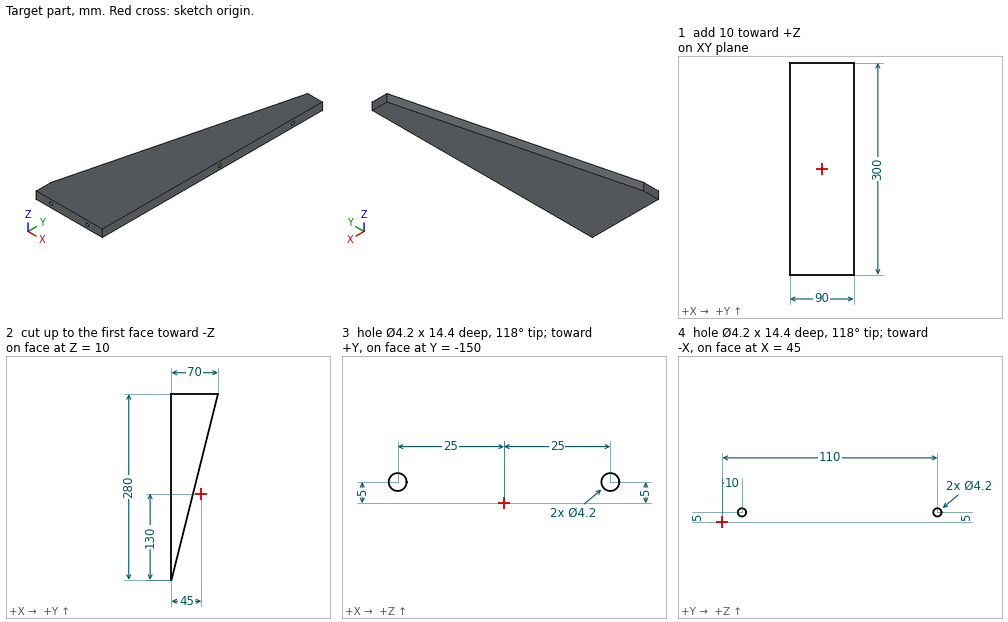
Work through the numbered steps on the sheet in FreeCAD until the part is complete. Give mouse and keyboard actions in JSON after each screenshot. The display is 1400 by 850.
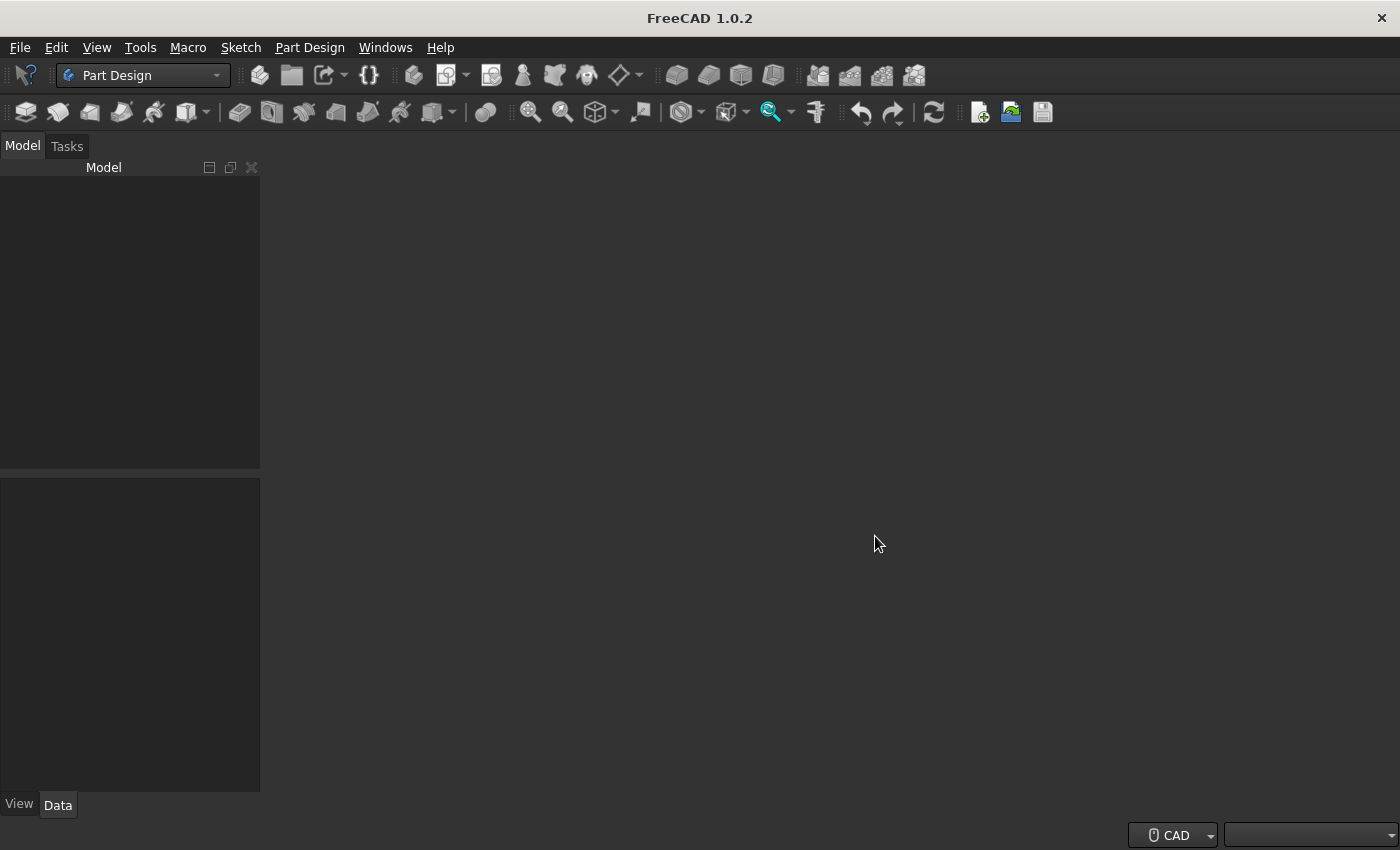
{"action": "key", "text": "ctrl+n"}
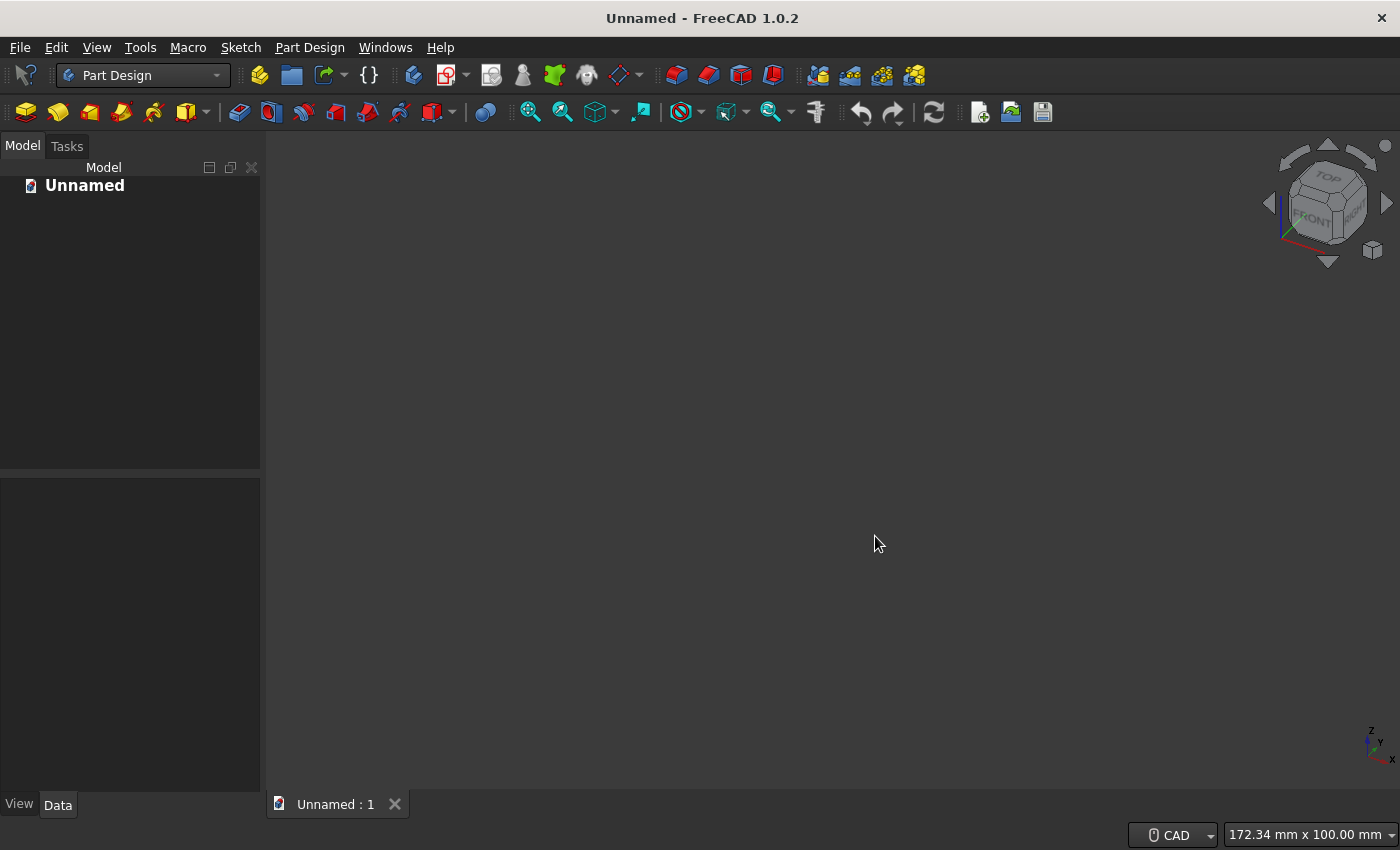
{"action": "left_click", "coordinate": [446, 76]}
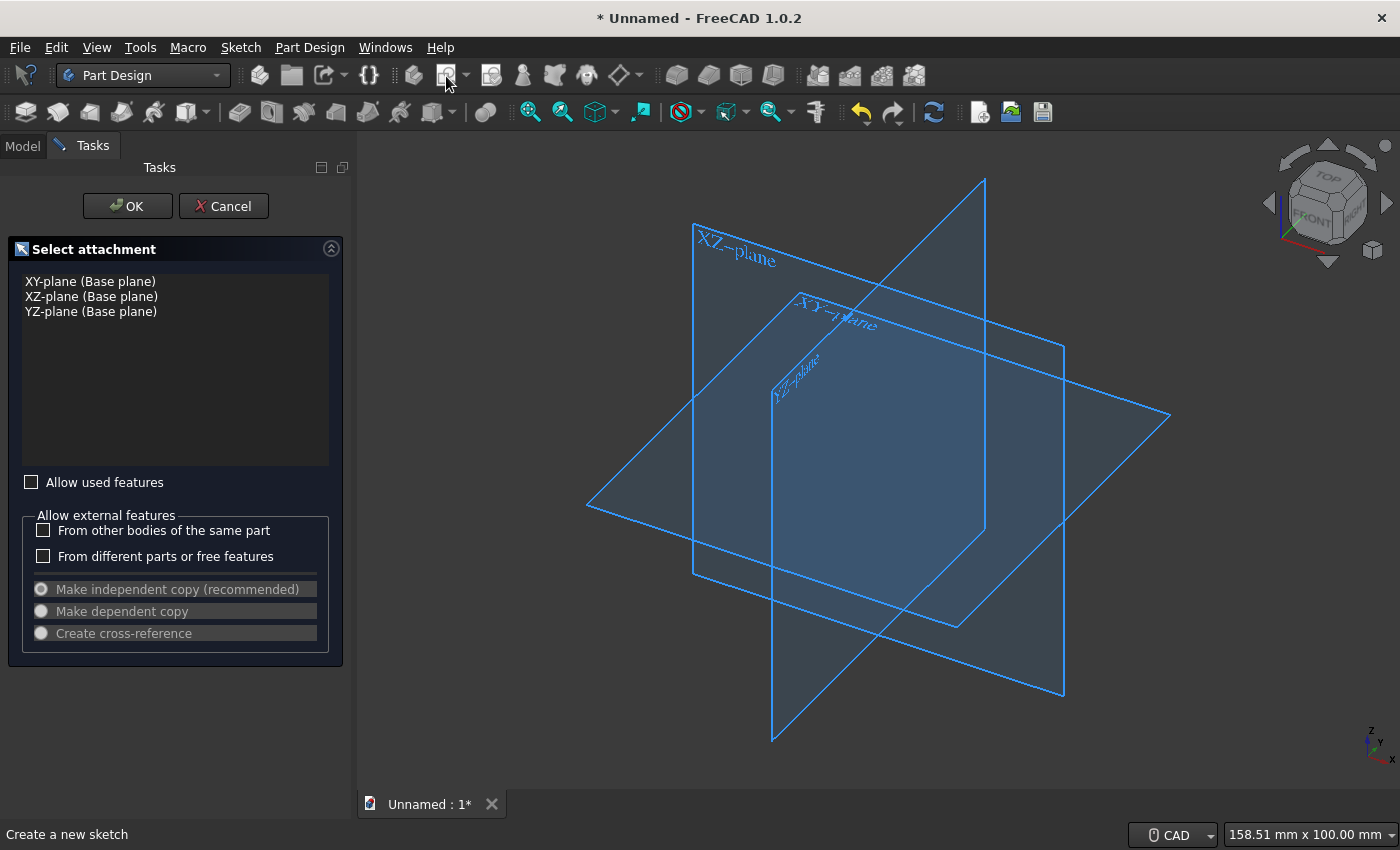
{"action": "left_click", "coordinate": [82, 282]}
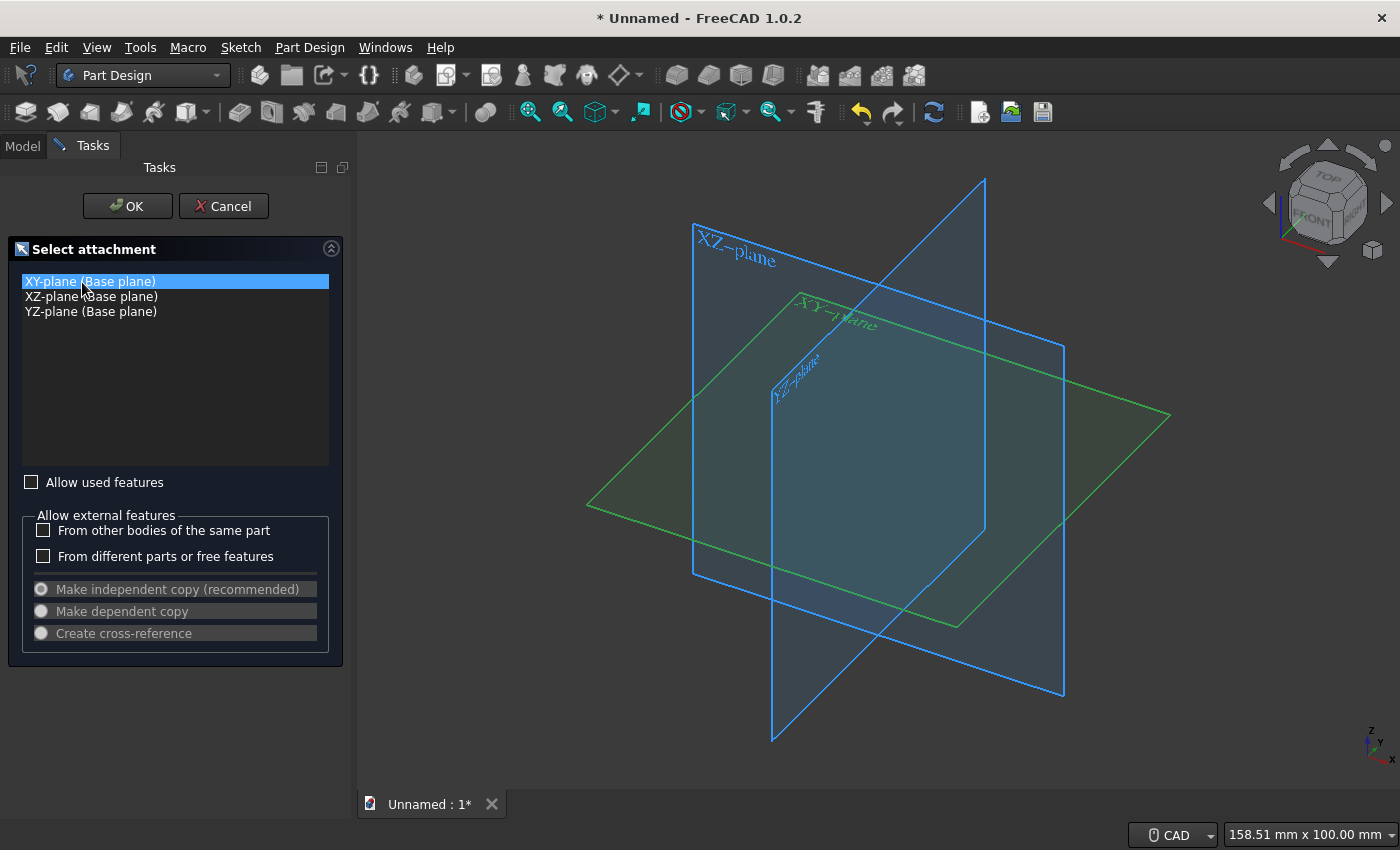
{"action": "left_click", "coordinate": [128, 206]}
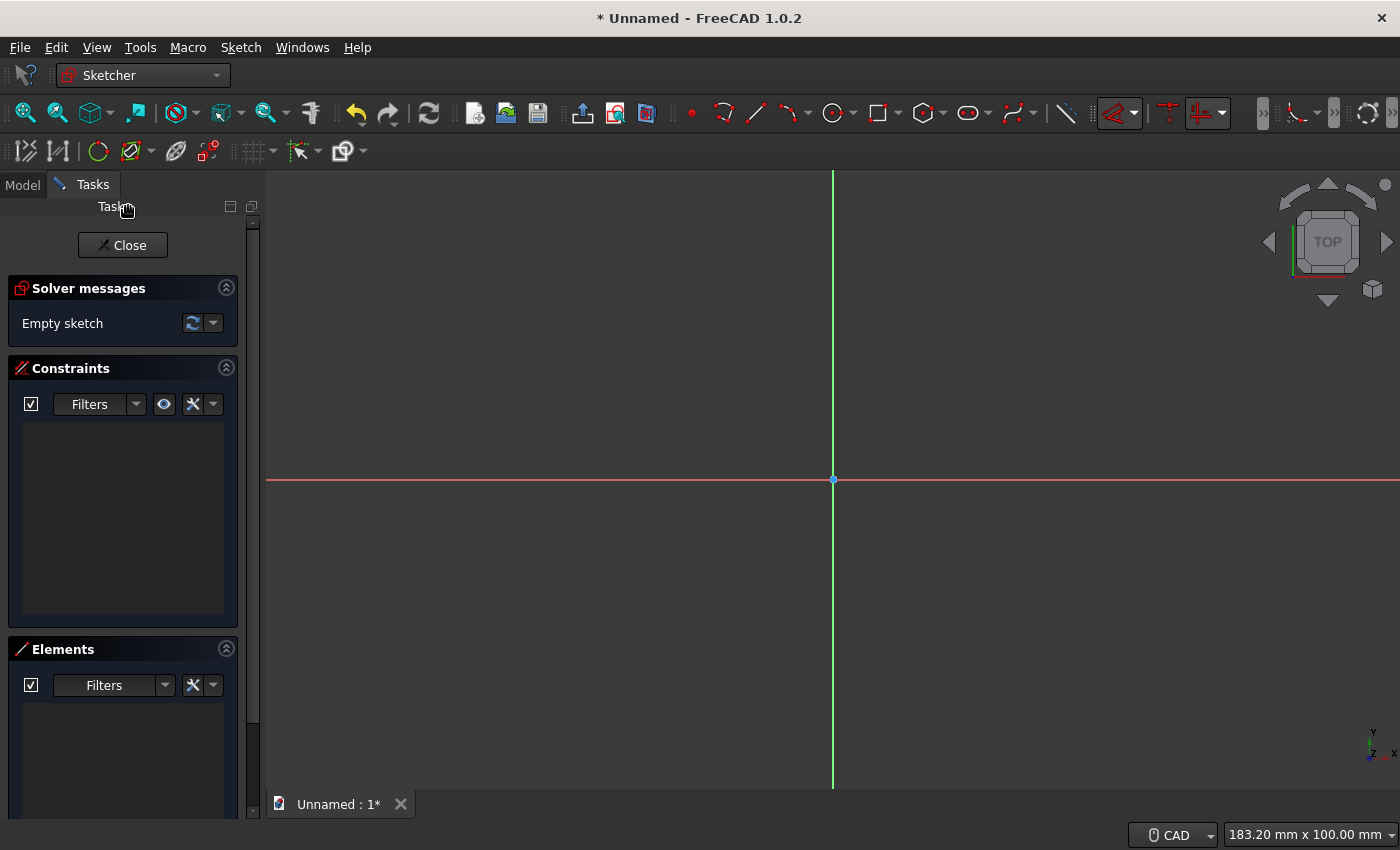
{"action": "scroll", "coordinate": [747, 480], "scroll_direction": "down", "scroll_amount": 8}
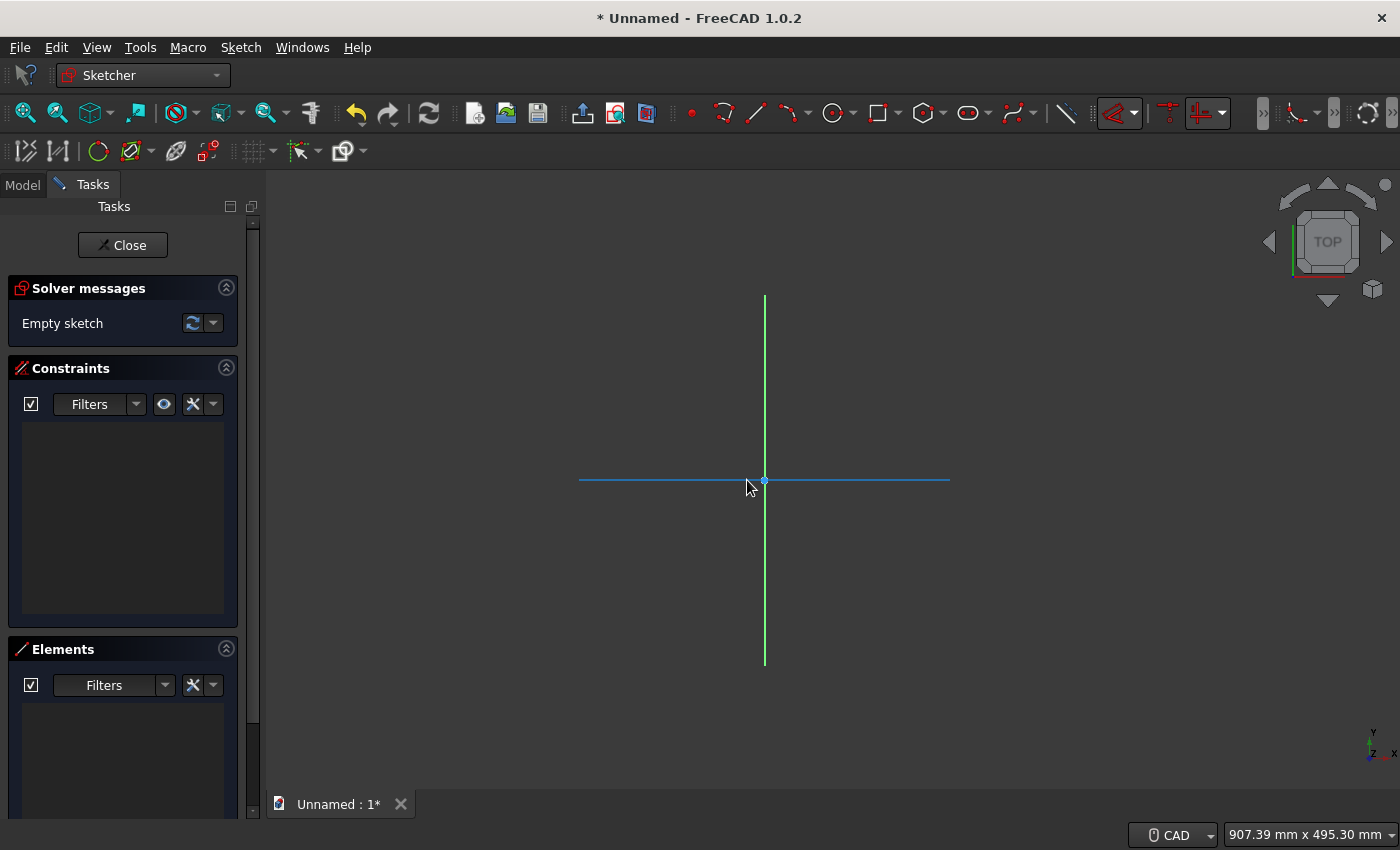
{"action": "key", "text": "g v"}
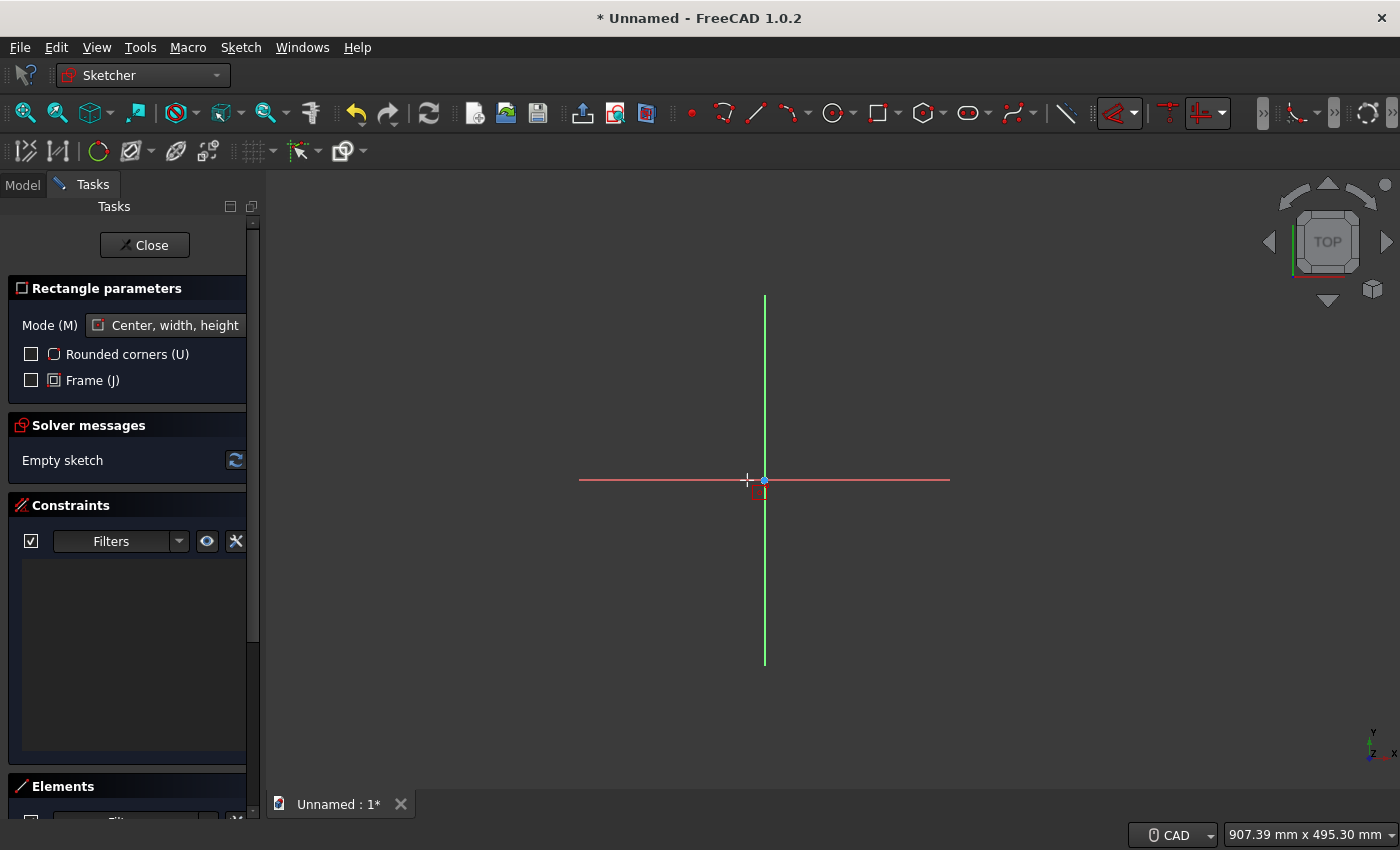
{"action": "left_click", "coordinate": [765, 480]}
{"action": "left_click", "coordinate": [821, 293]}
{"action": "key", "text": "Escape"}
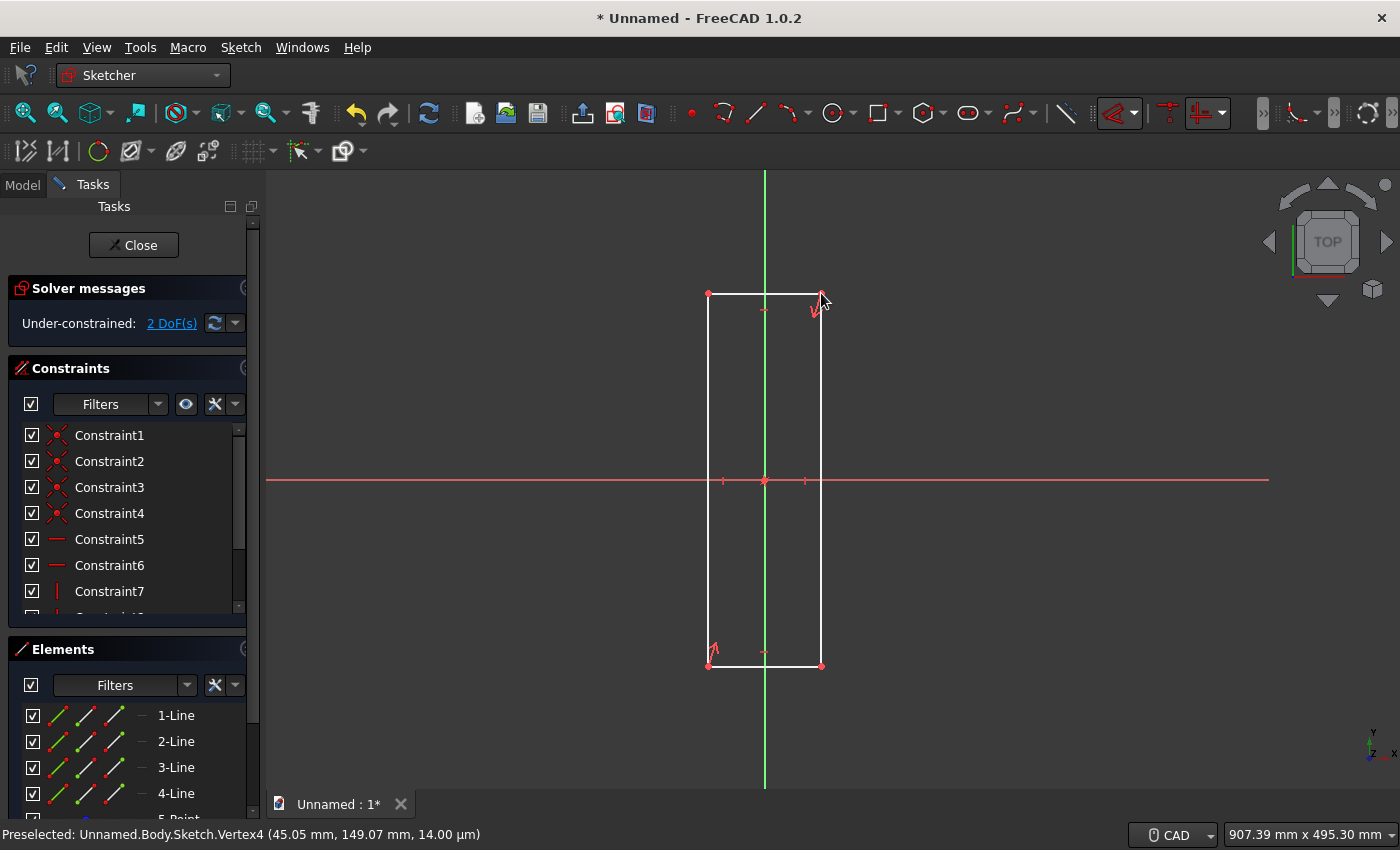
{"action": "left_click", "coordinate": [1114, 114]}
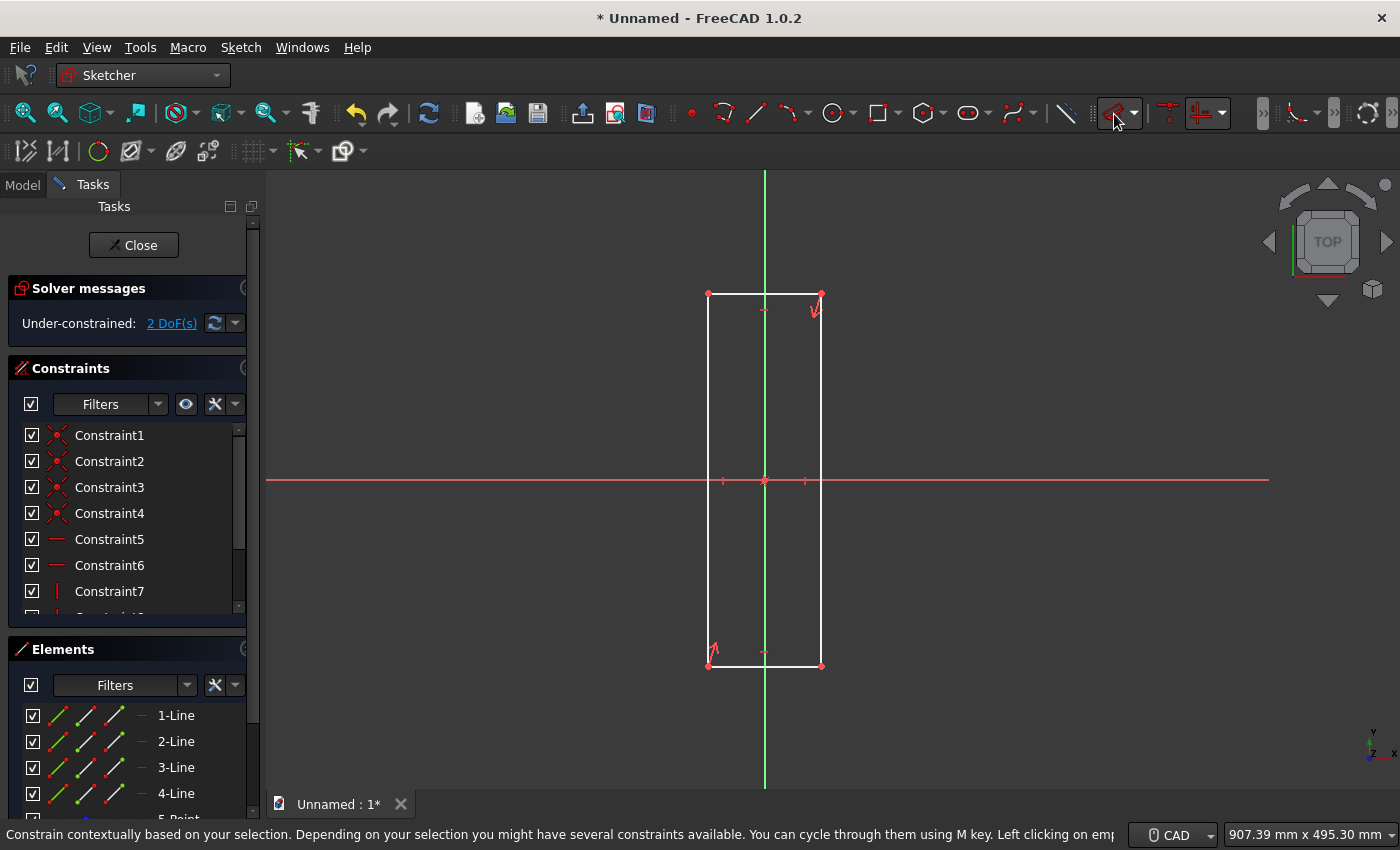
{"action": "left_click", "coordinate": [742, 667]}
{"action": "left_click", "coordinate": [739, 701]}